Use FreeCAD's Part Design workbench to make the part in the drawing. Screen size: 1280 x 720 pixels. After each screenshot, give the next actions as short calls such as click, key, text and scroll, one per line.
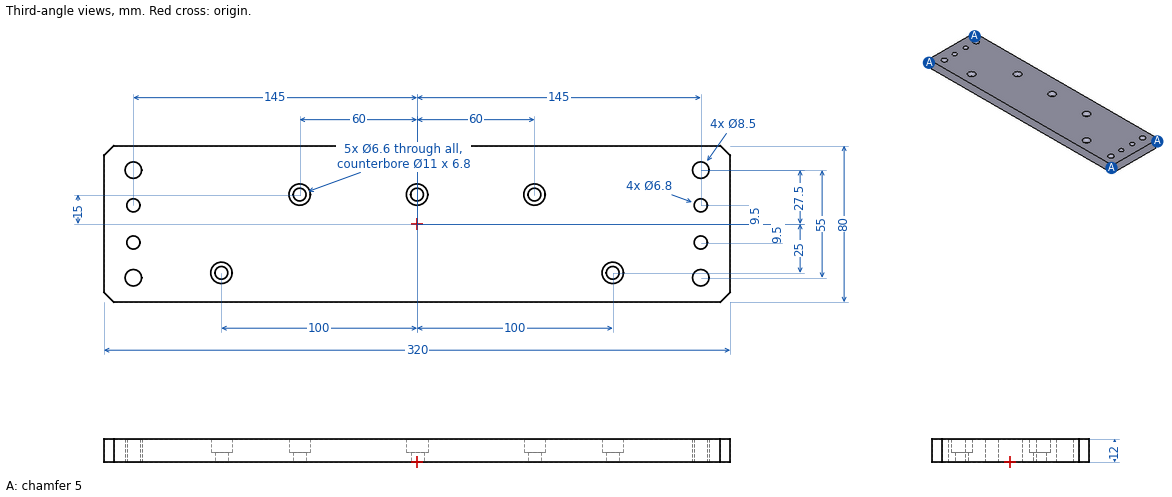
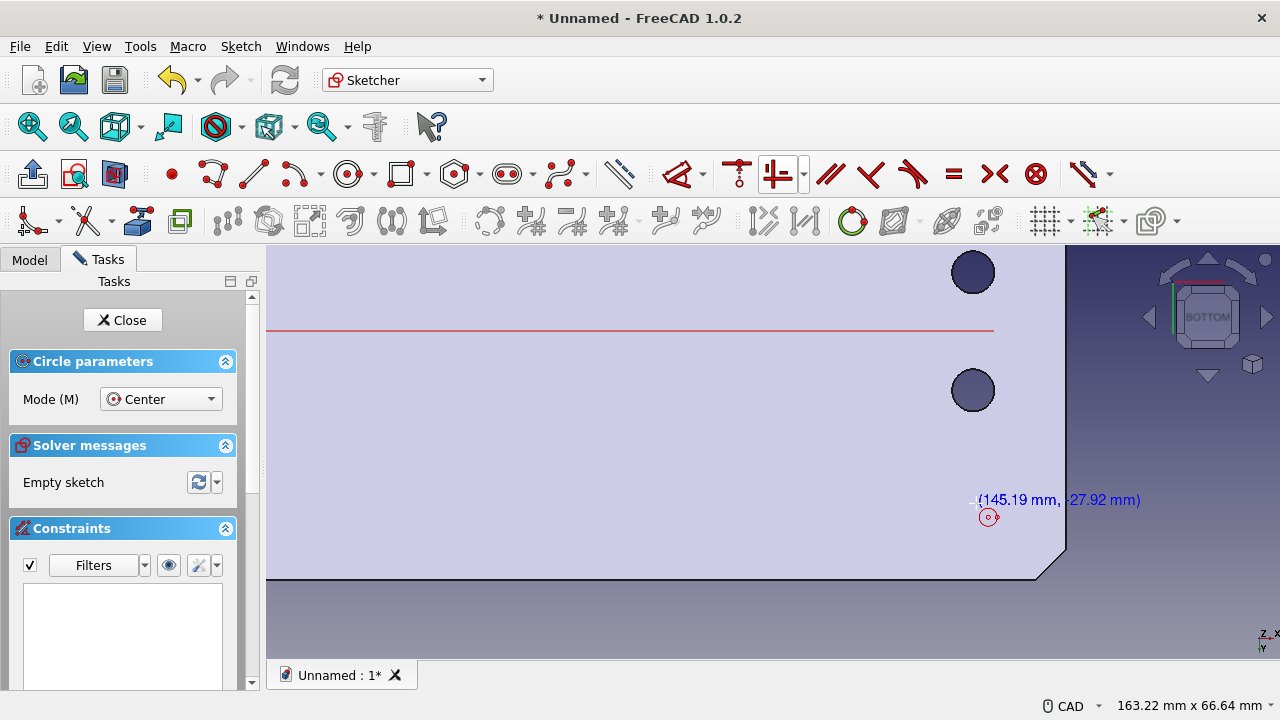
click(973, 502)
click(992, 484)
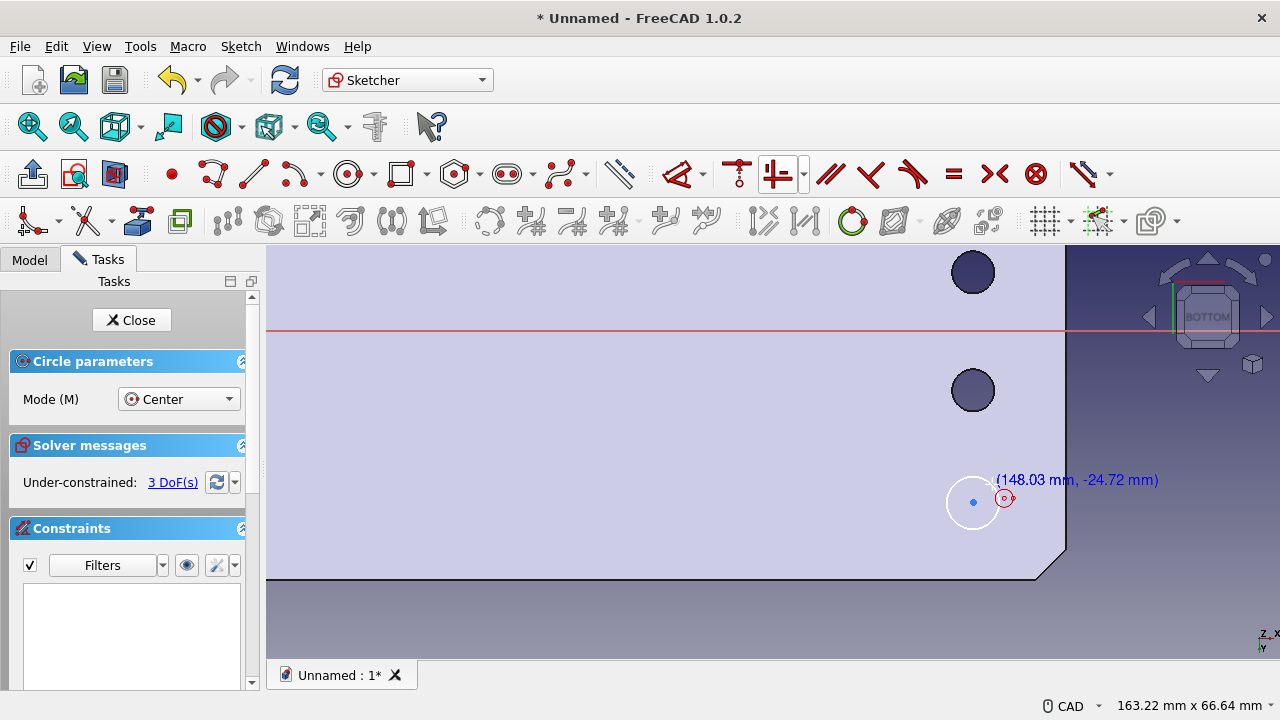
scroll(977, 504, down, 6)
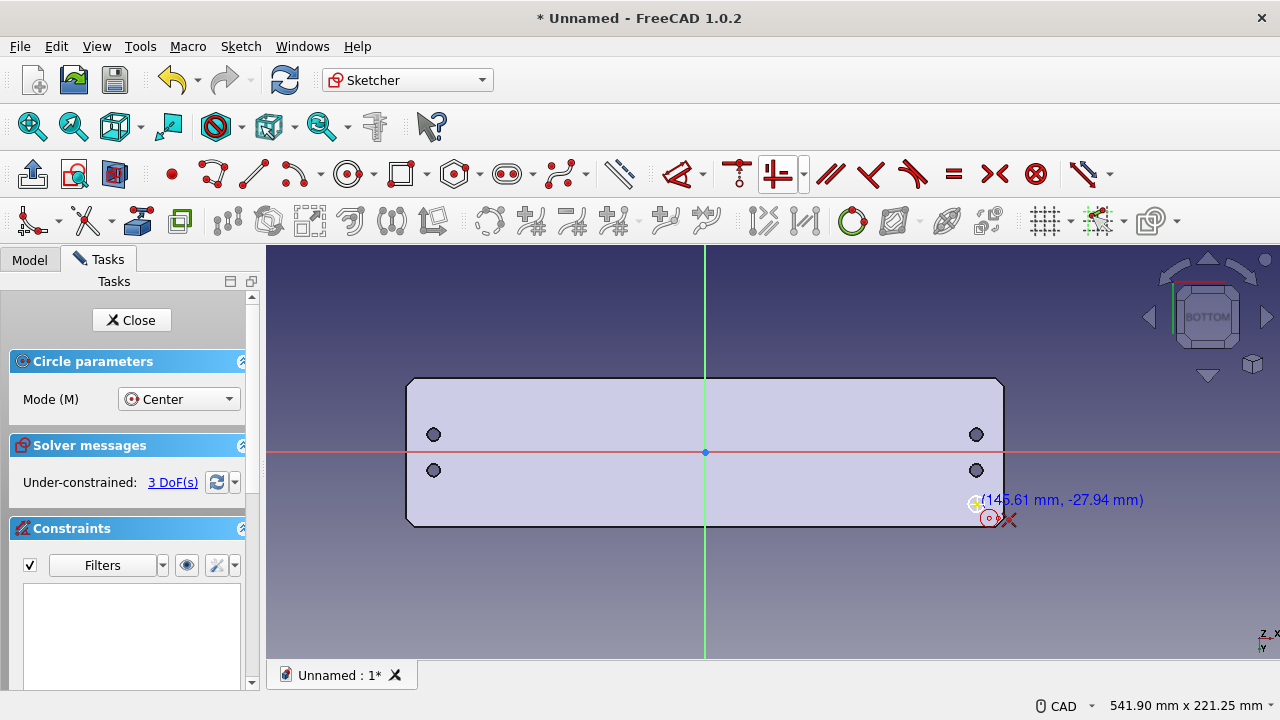
scroll(976, 401, up, 6)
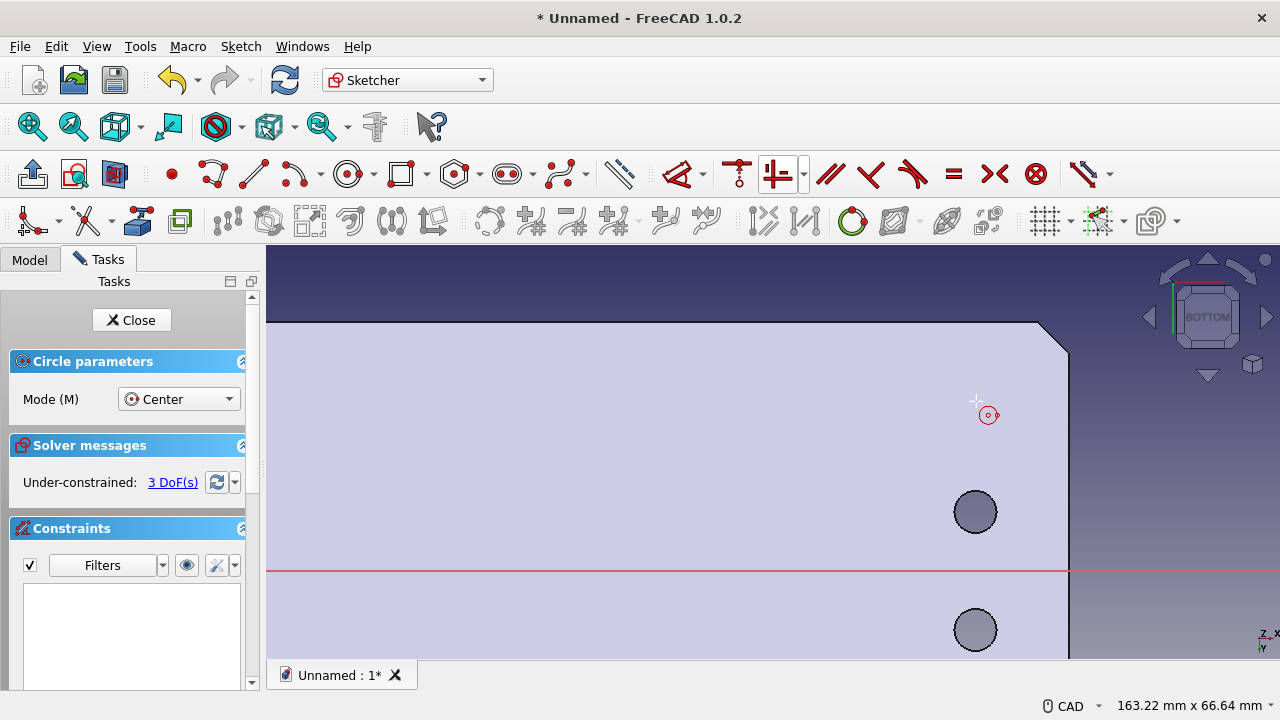
click(976, 400)
click(994, 381)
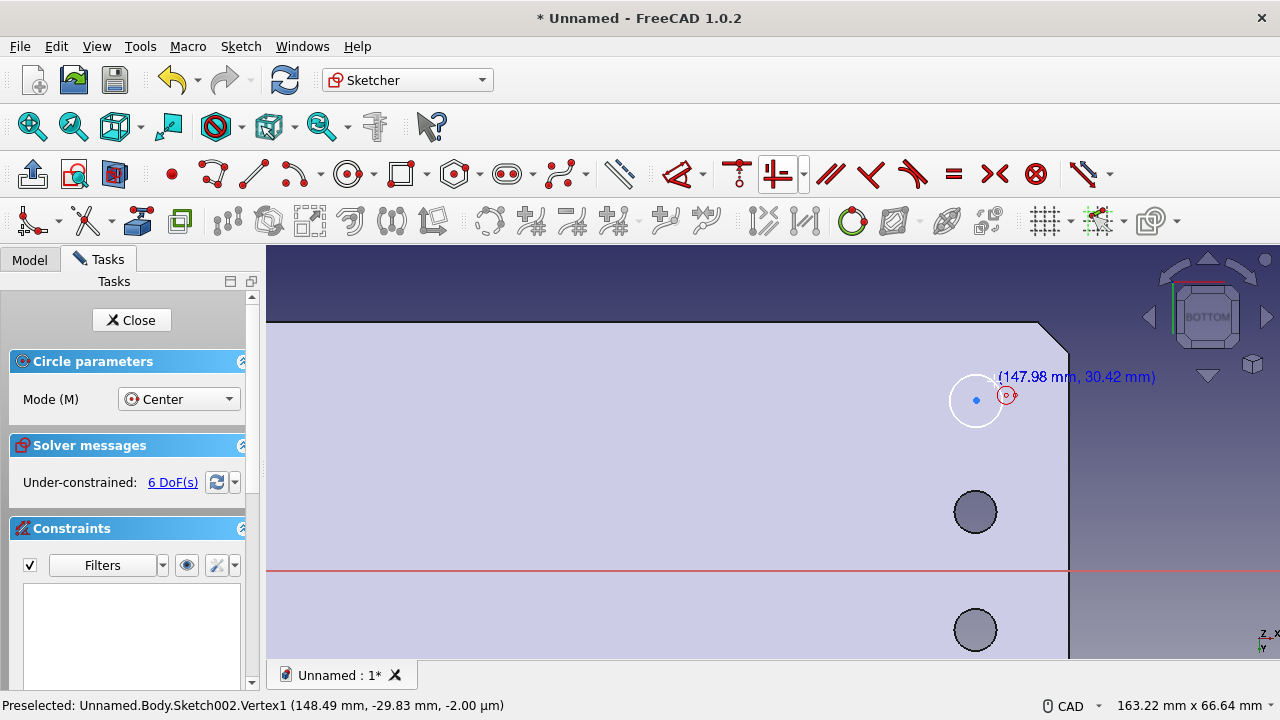
scroll(976, 401, down, 6)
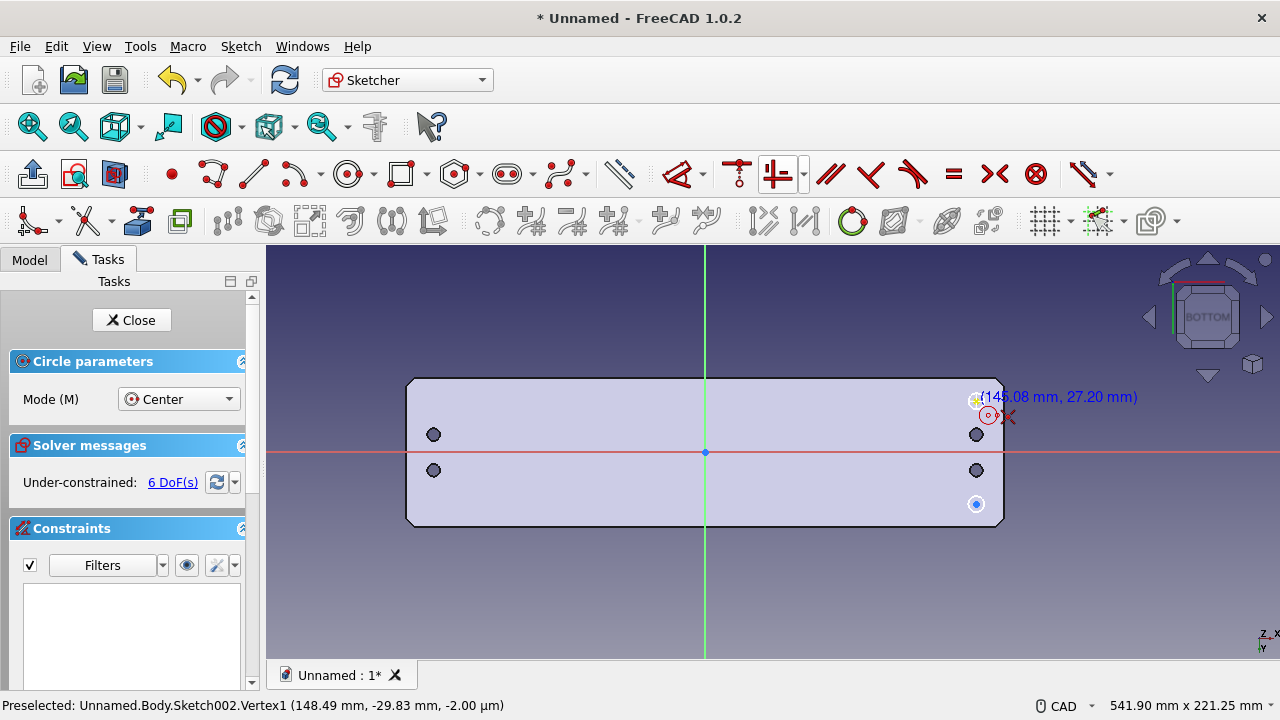
scroll(434, 504, up, 6)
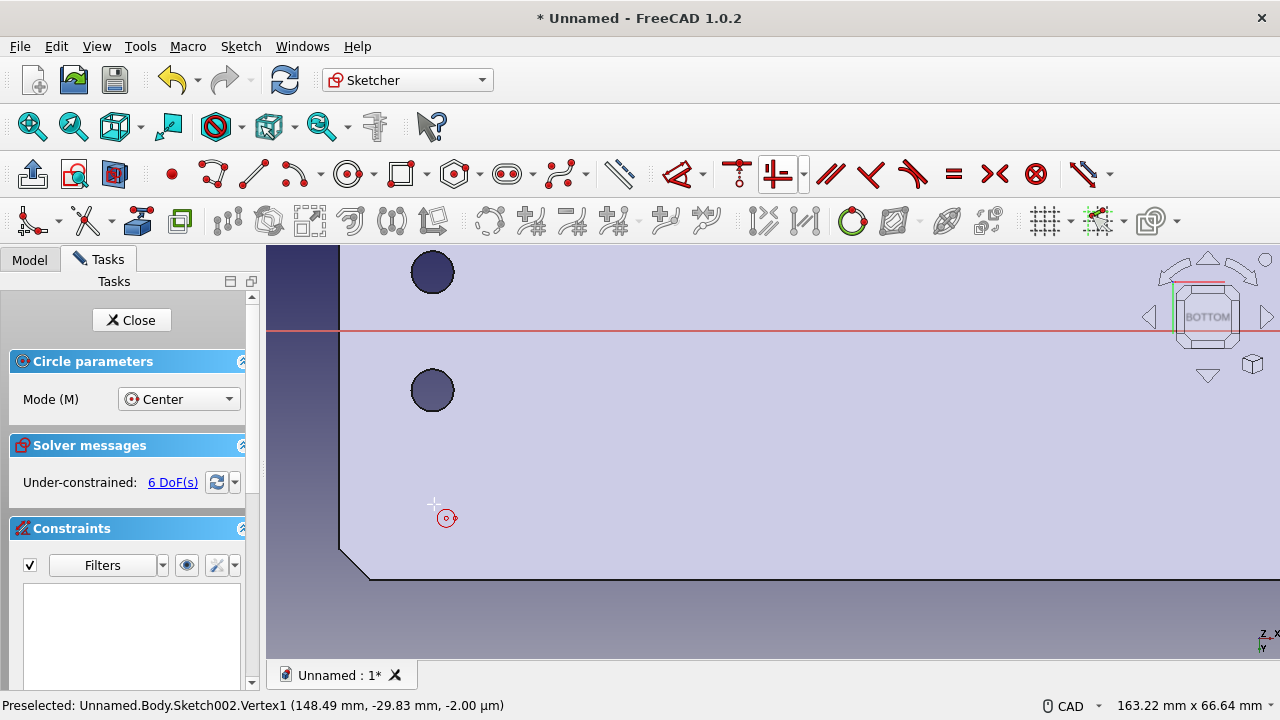
click(433, 502)
click(451, 484)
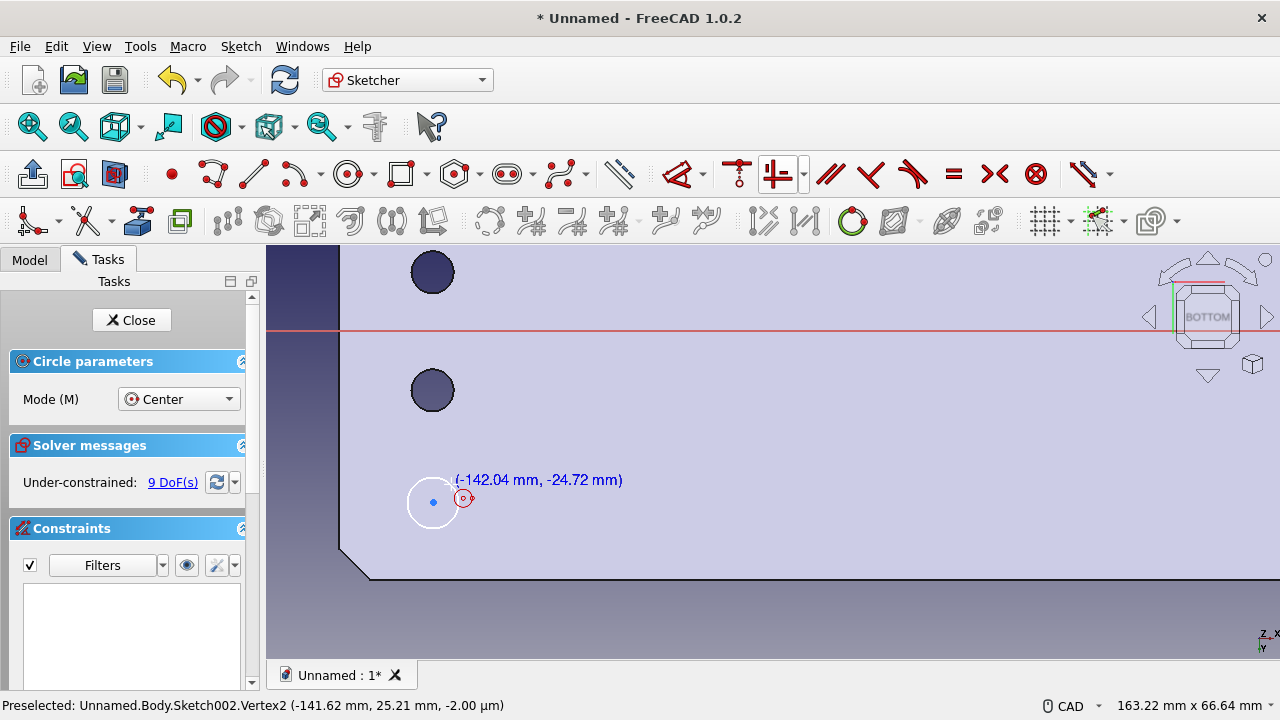
scroll(433, 504, down, 6)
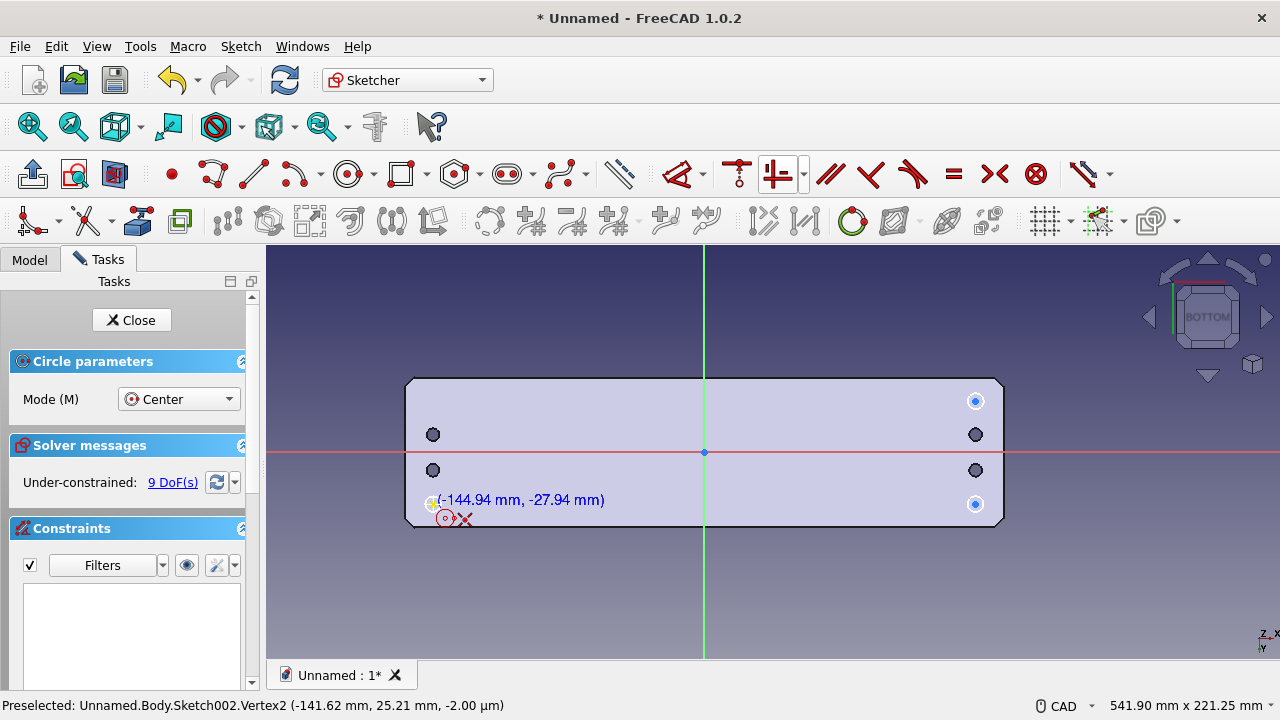
scroll(433, 401, up, 6)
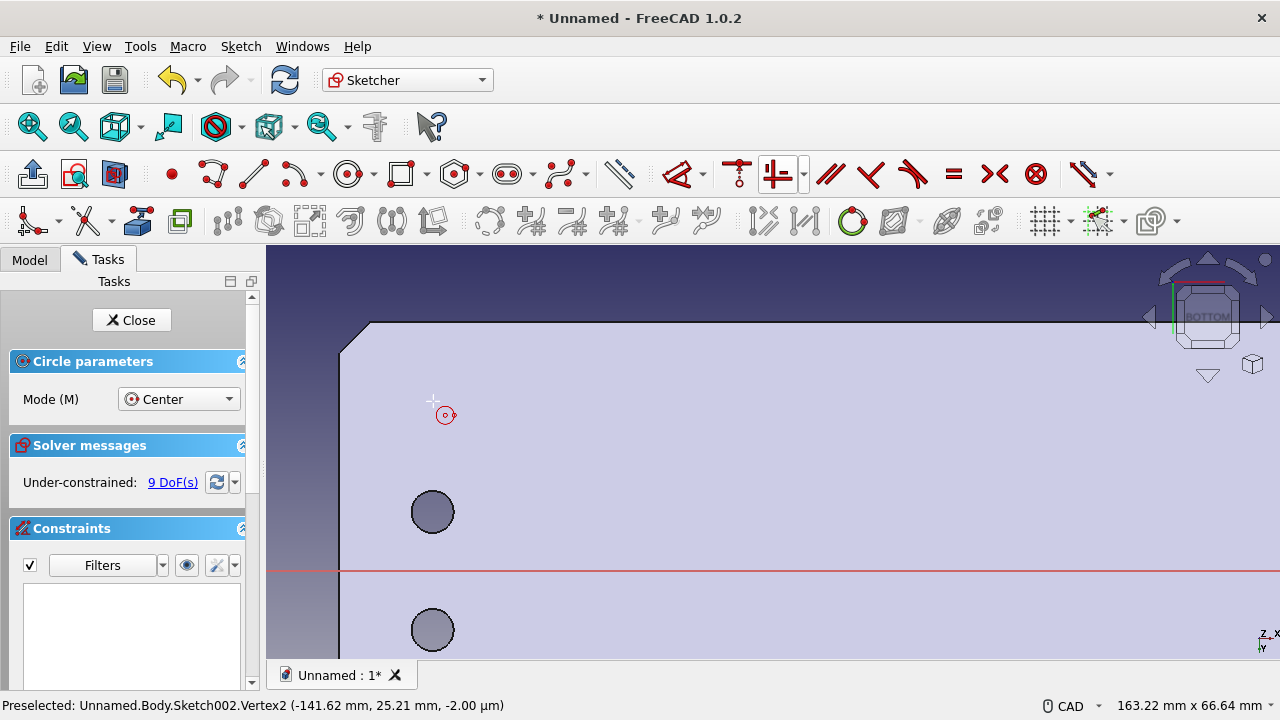
click(433, 400)
click(451, 381)
key(Escape)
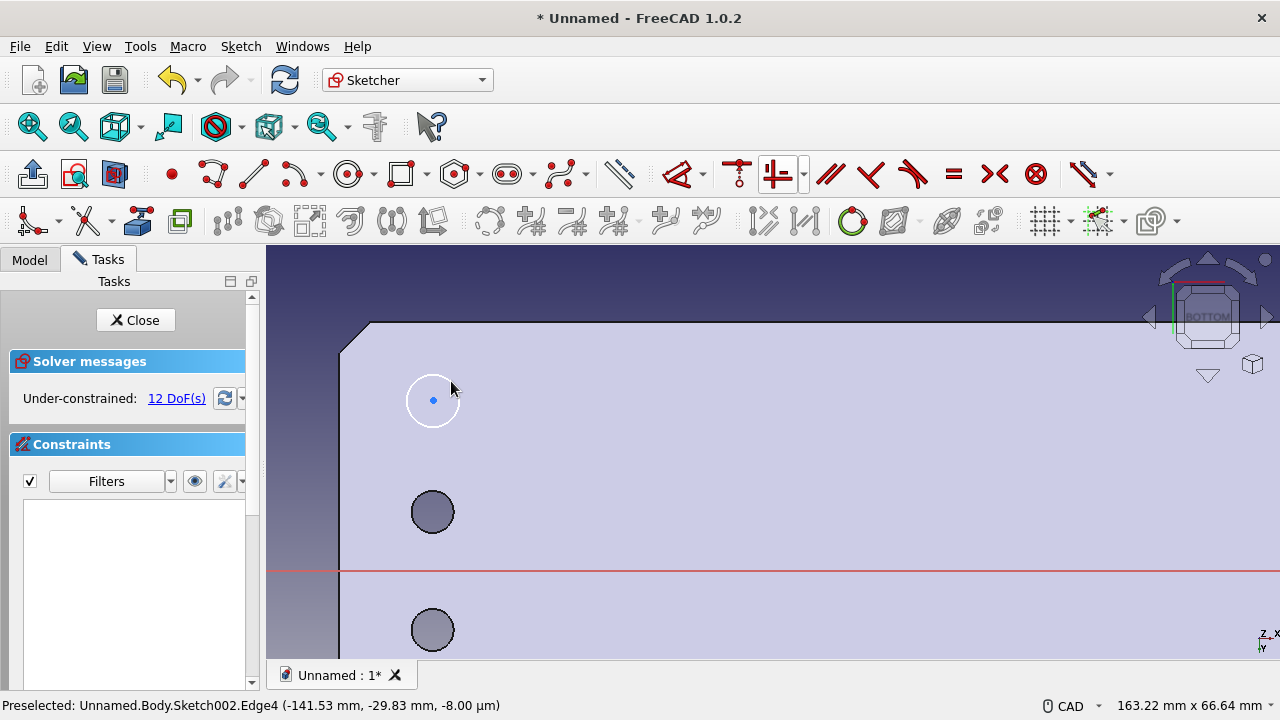
scroll(433, 401, down, 6)